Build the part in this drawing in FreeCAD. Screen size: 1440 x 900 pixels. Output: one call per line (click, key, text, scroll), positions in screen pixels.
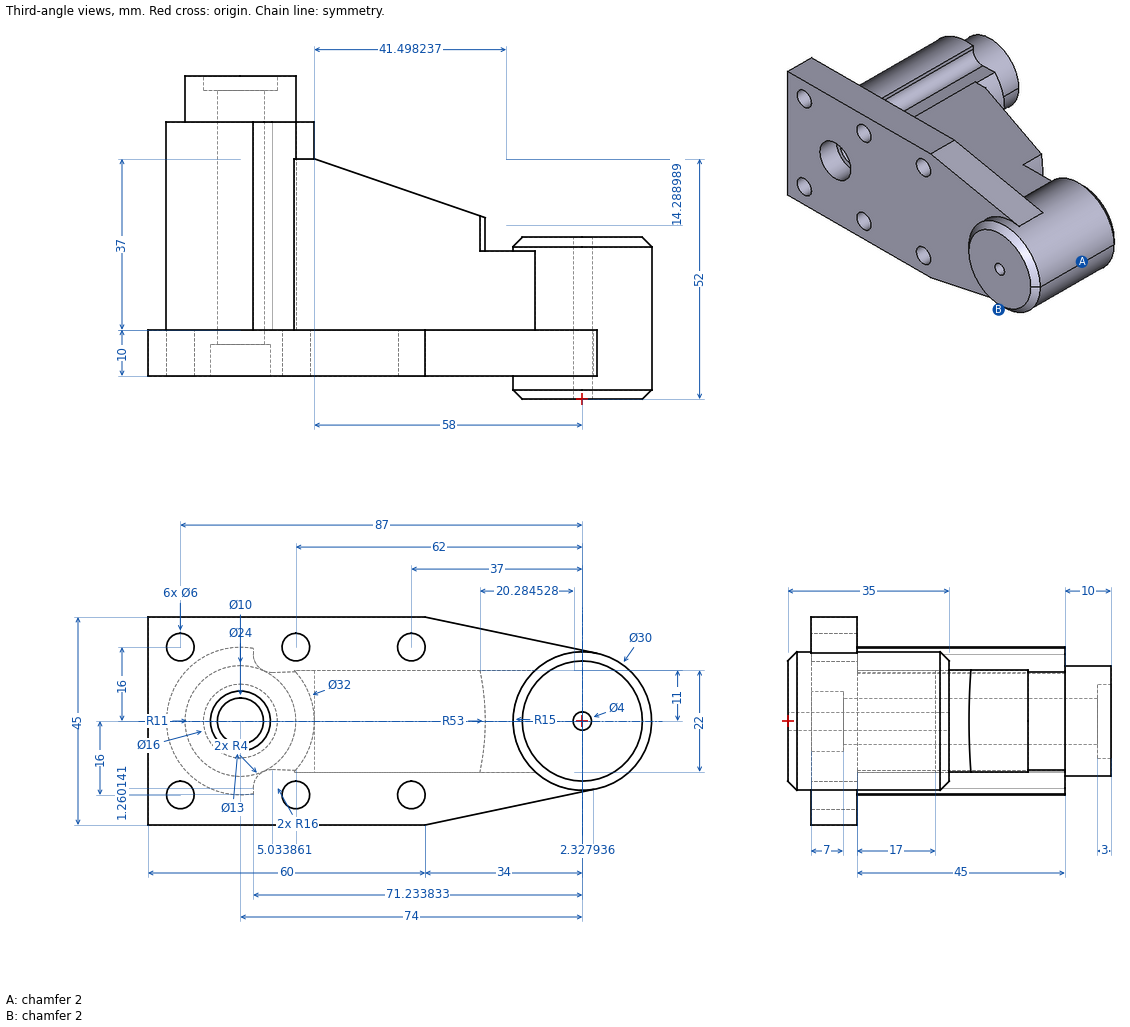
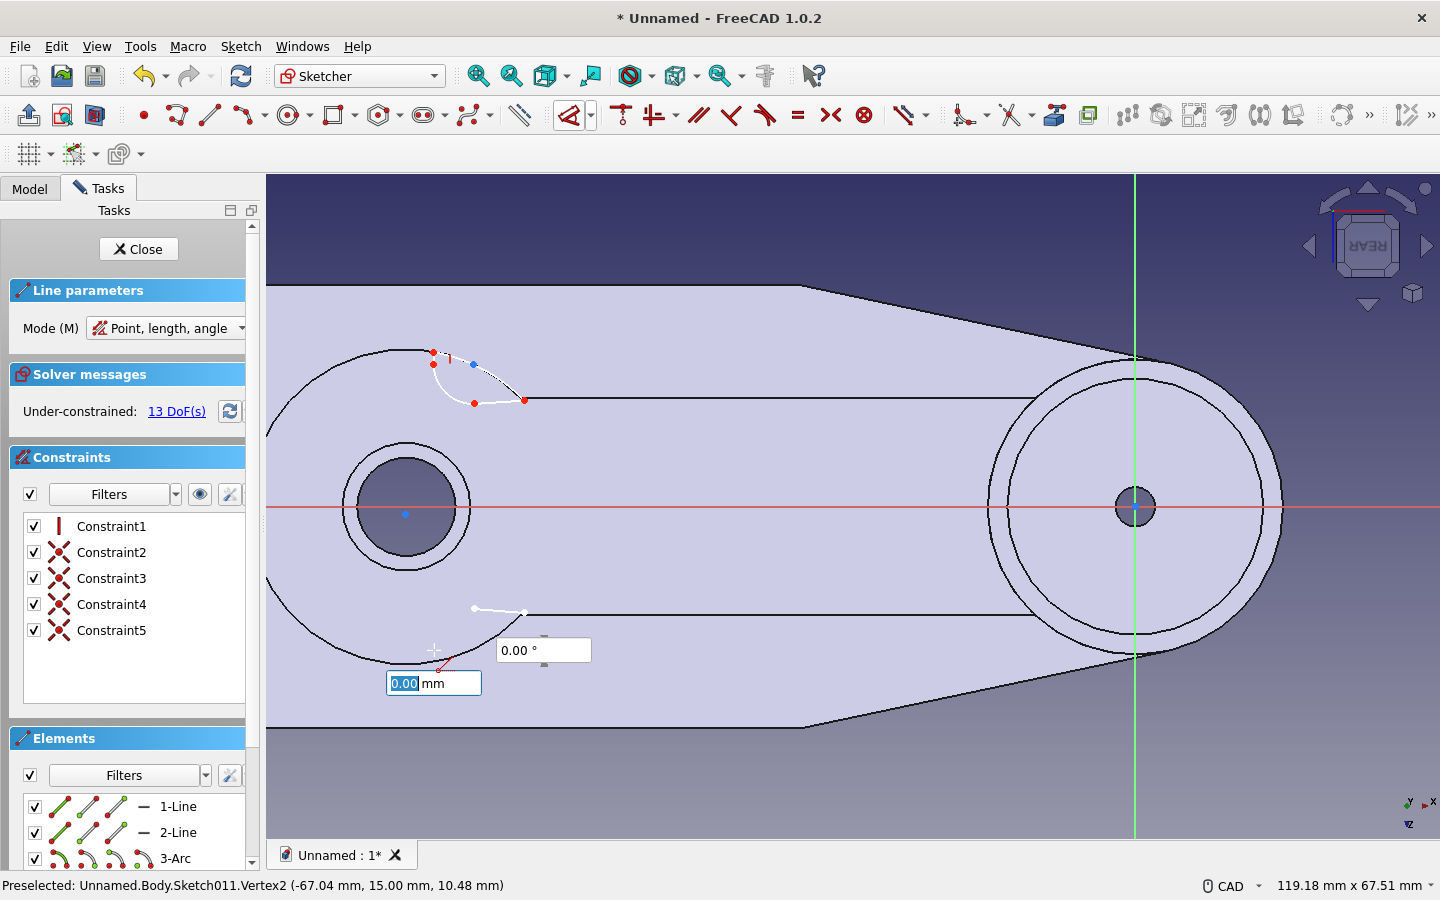
scroll(434, 662, up, 2)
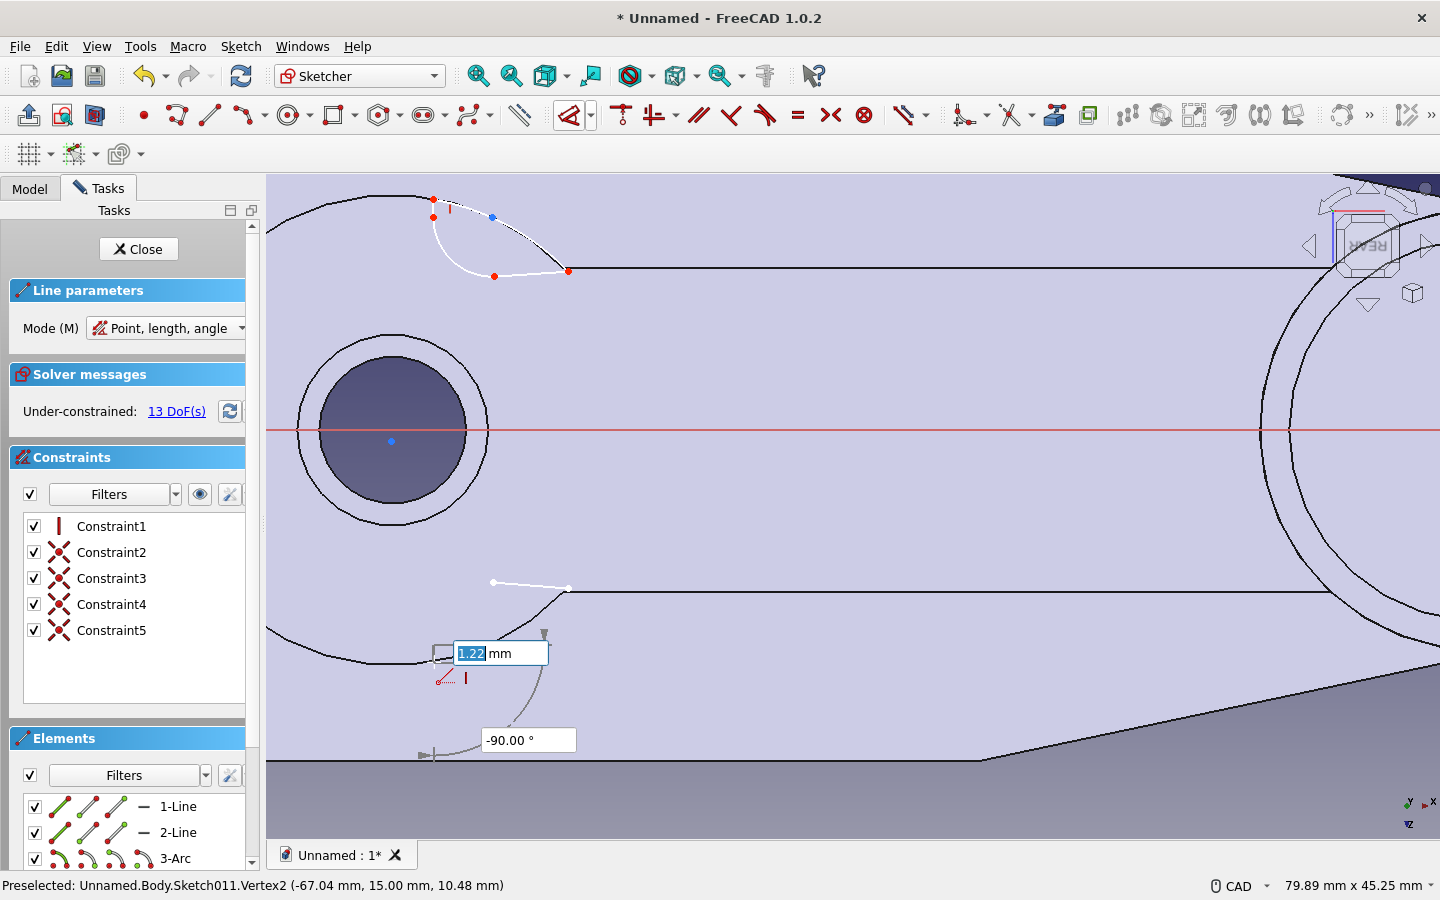
click(434, 662)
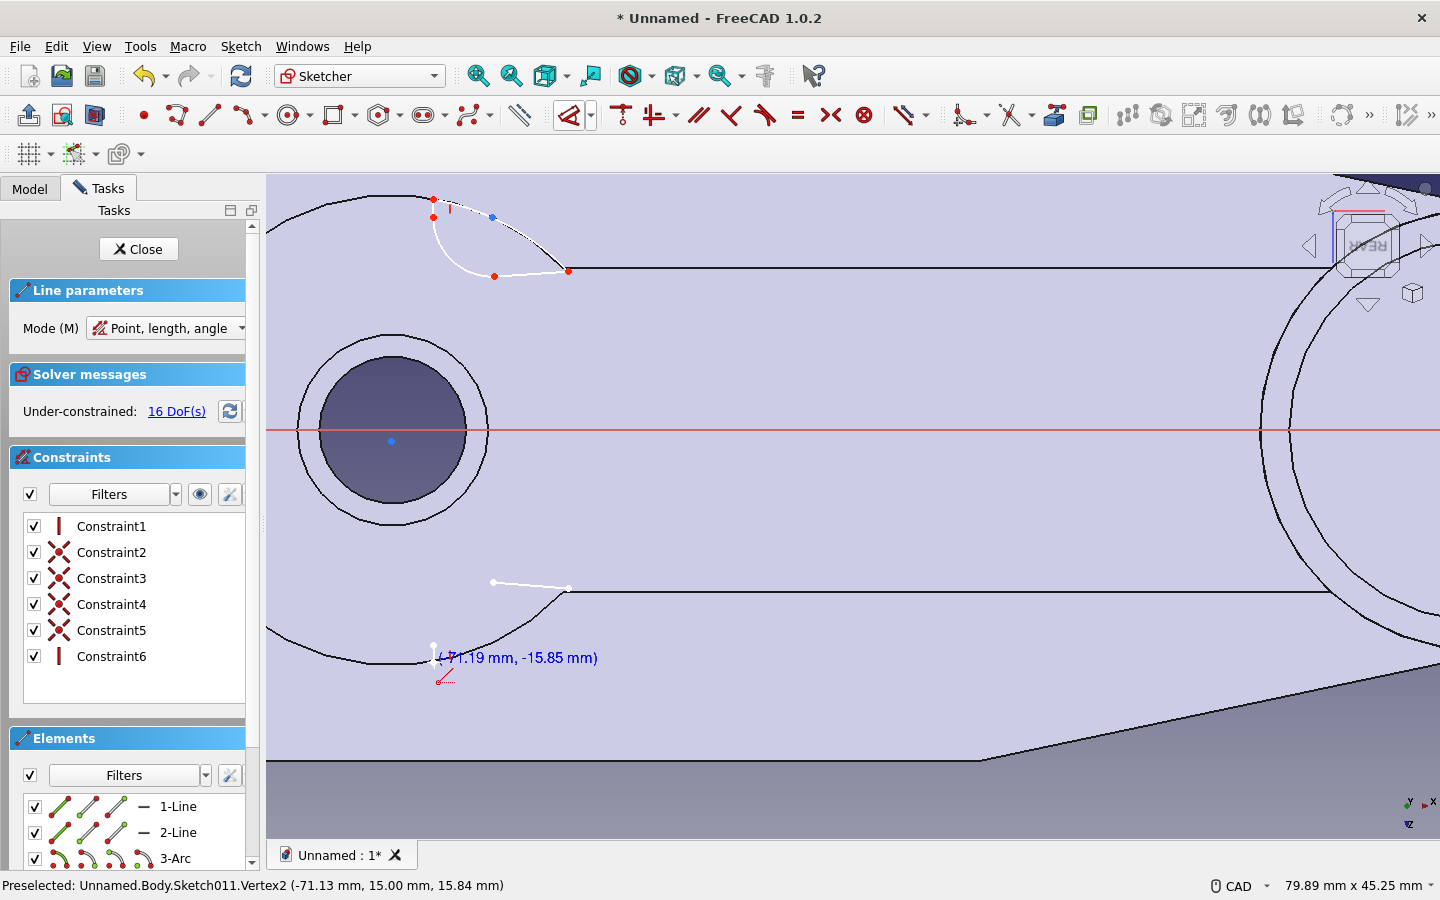
click(242, 116)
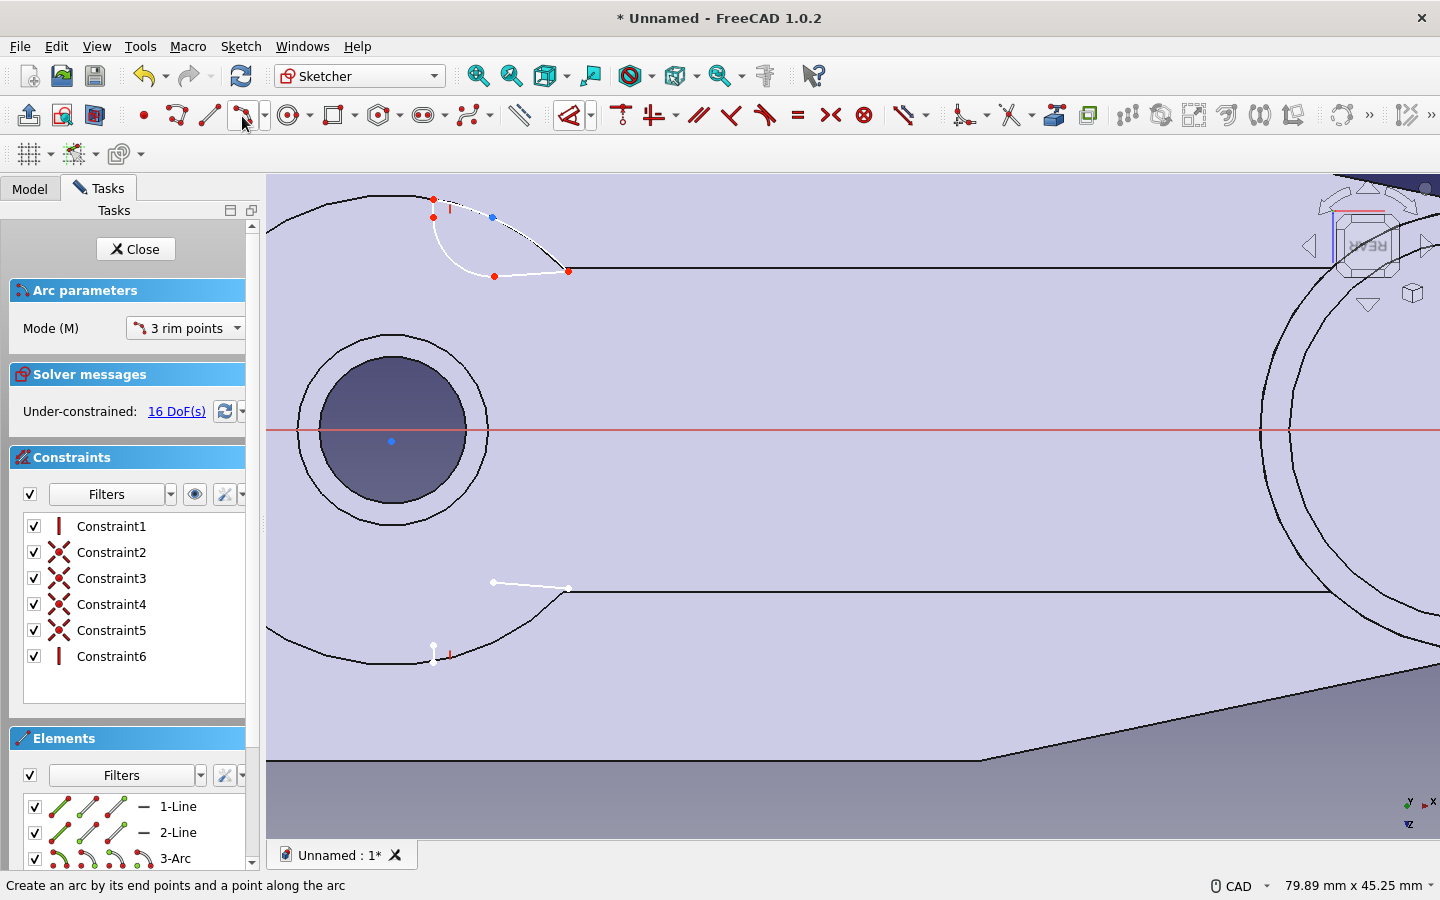
click(494, 583)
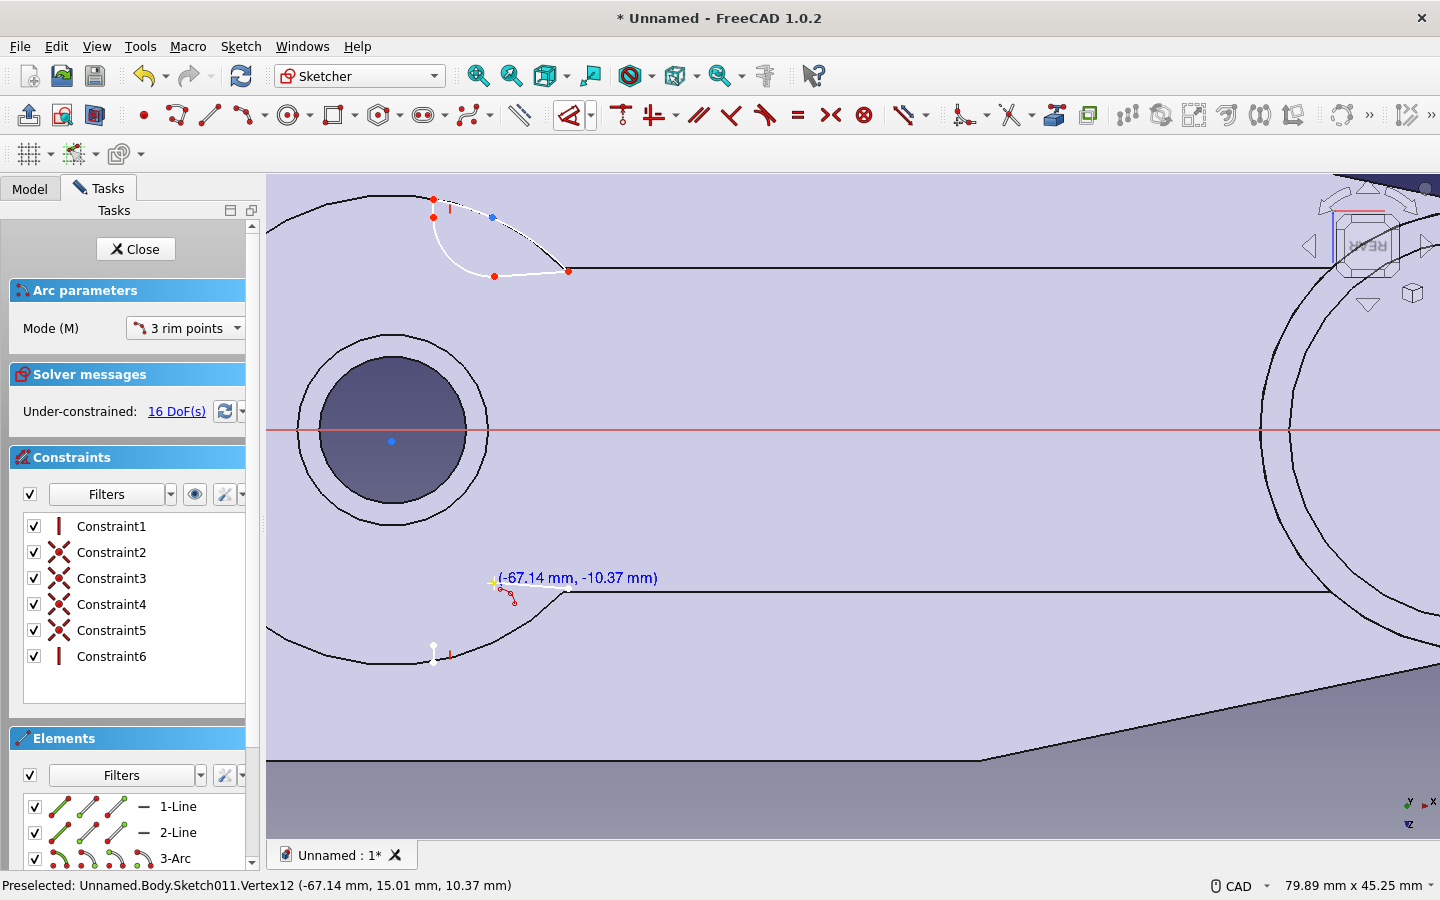
scroll(433, 643, up, 3)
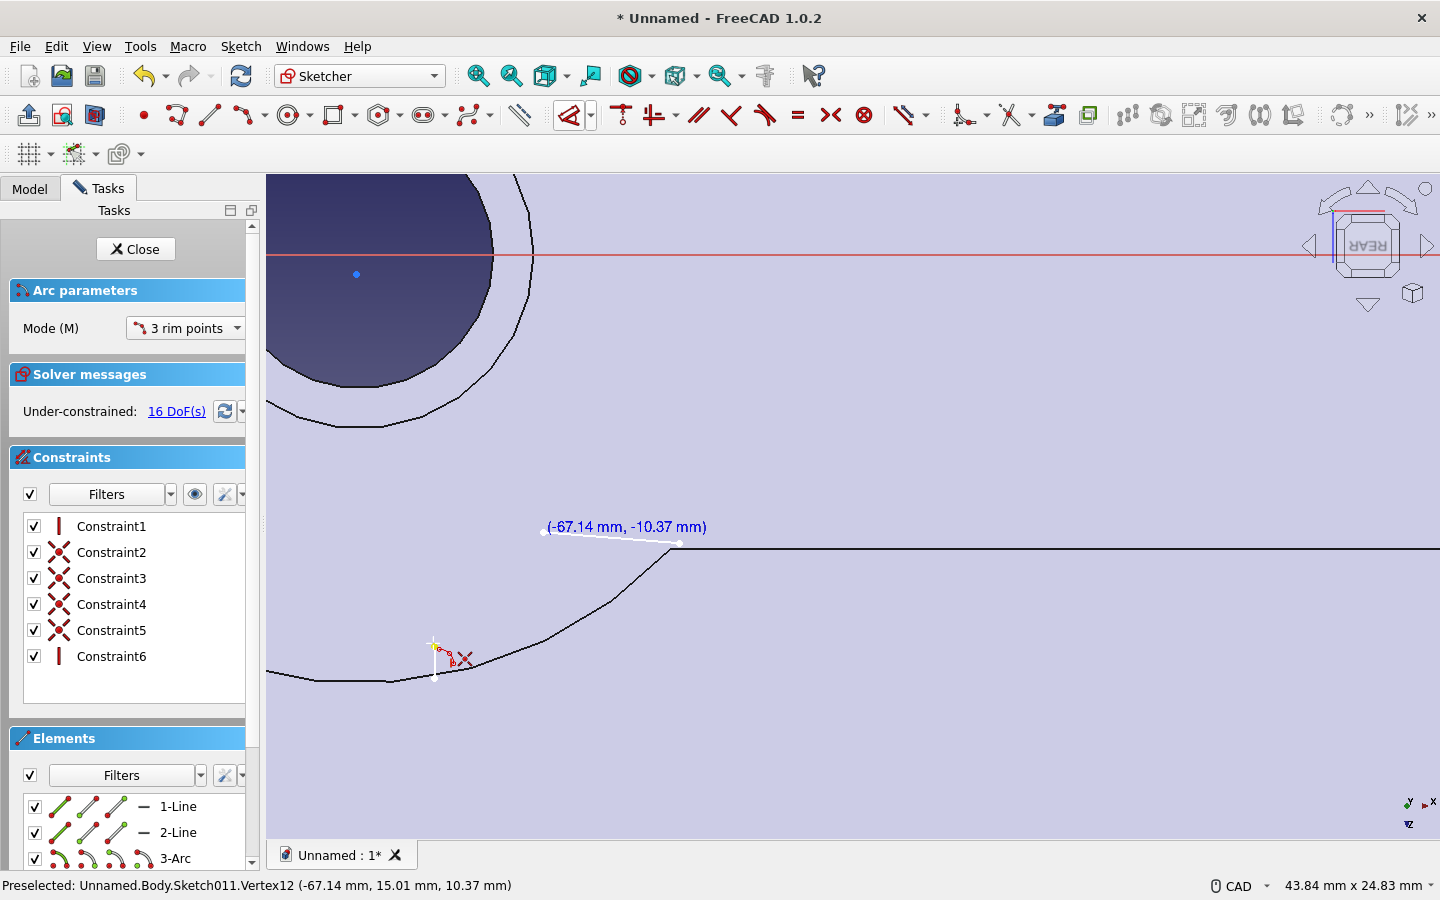
click(435, 646)
click(466, 566)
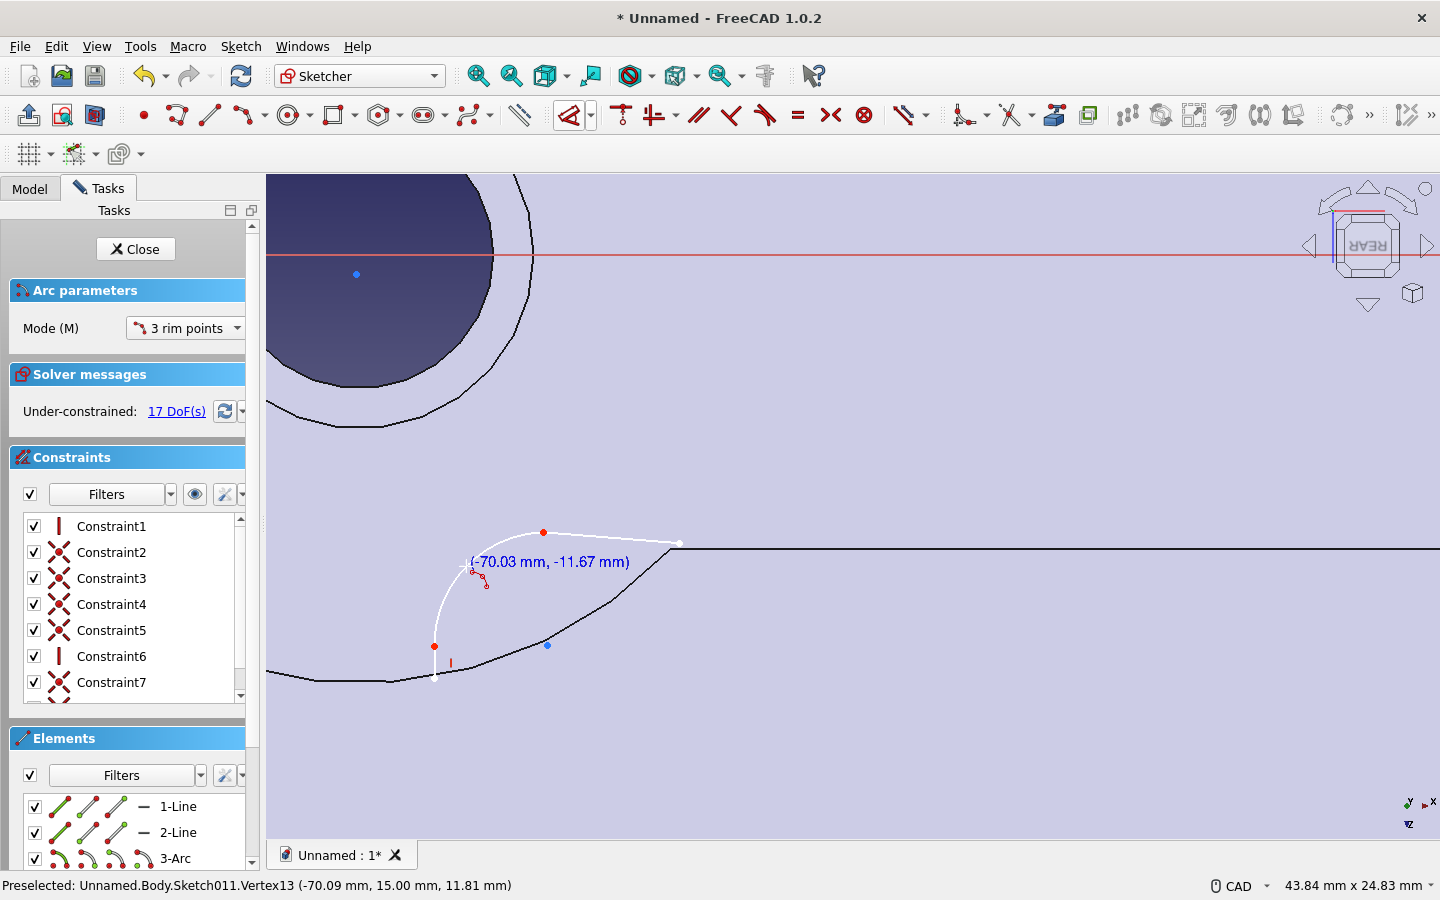
click(435, 679)
click(679, 543)
click(568, 629)
key(Escape)